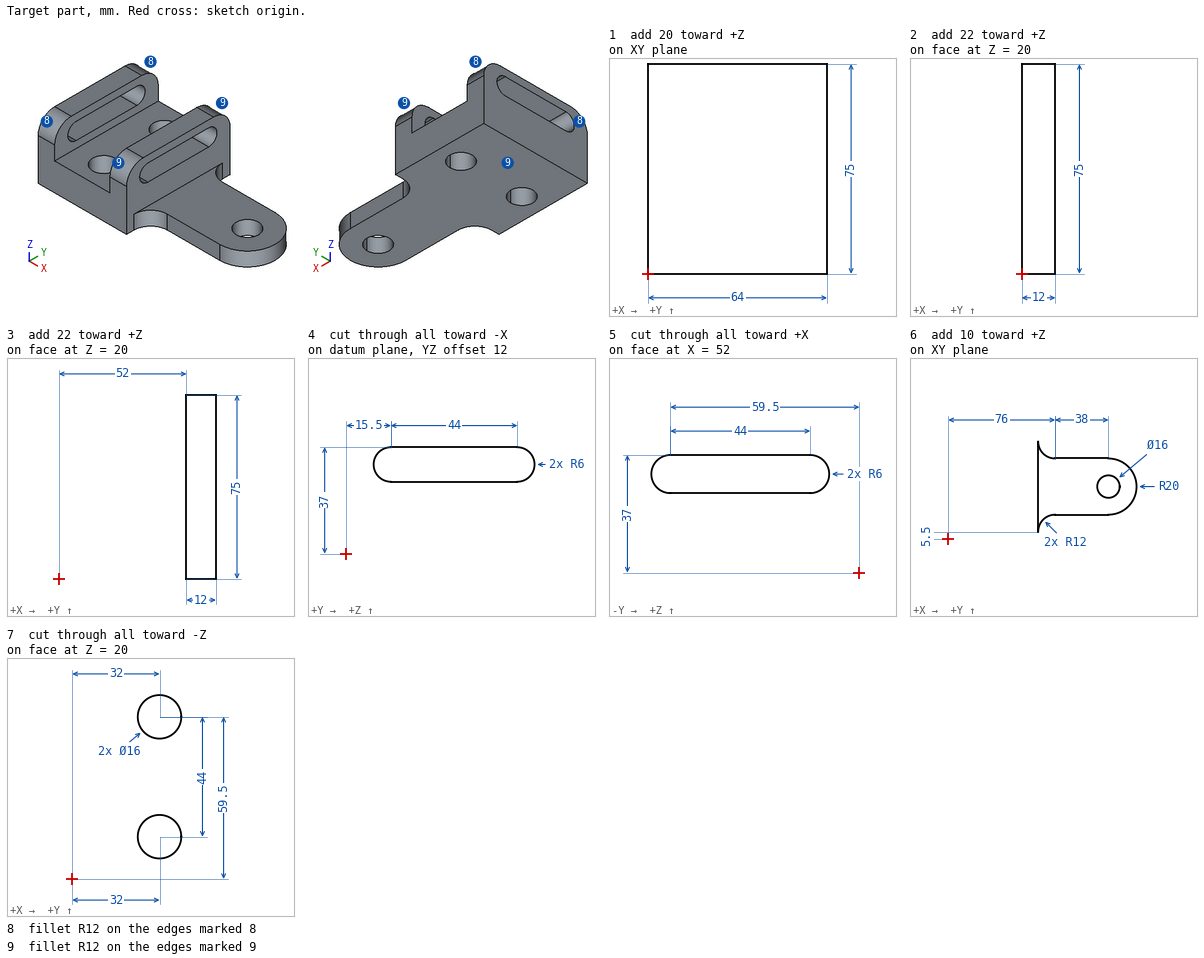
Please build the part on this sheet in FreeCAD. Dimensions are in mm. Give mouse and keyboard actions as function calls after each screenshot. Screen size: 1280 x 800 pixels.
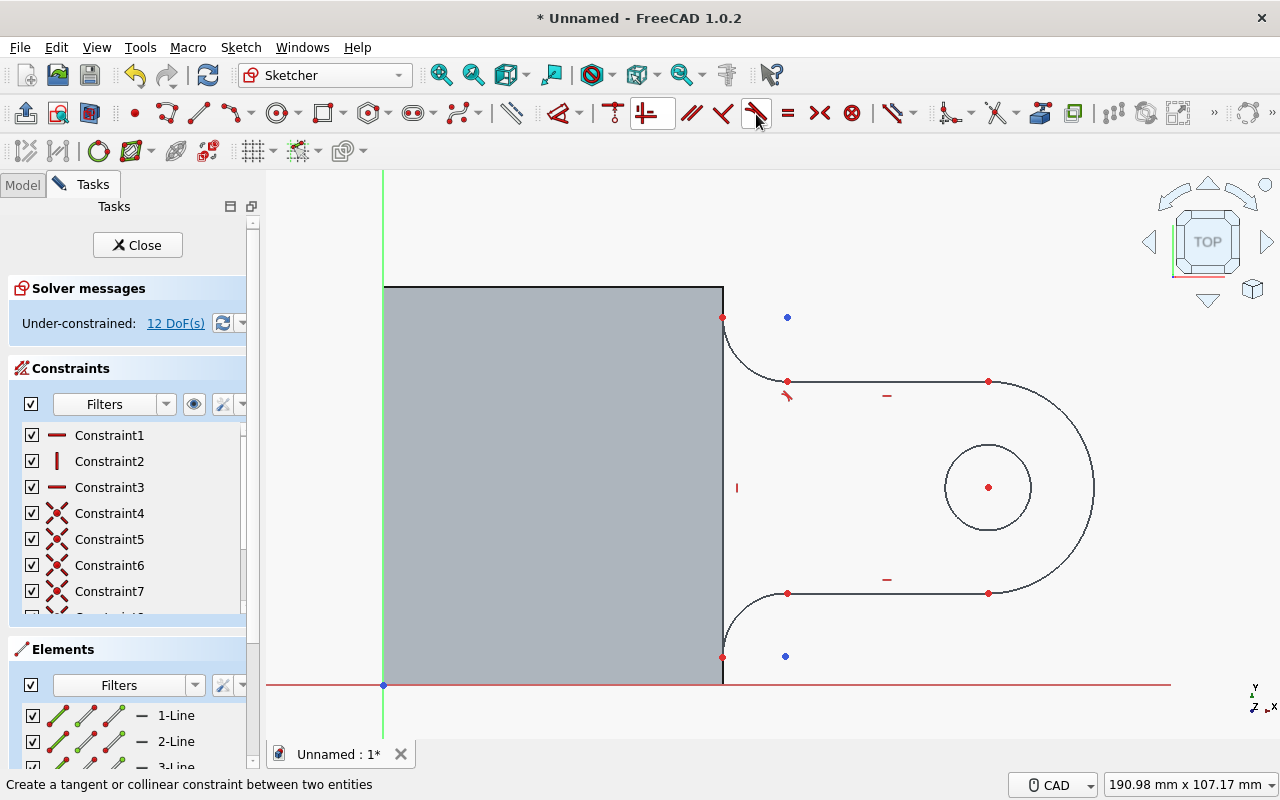
click(928, 382)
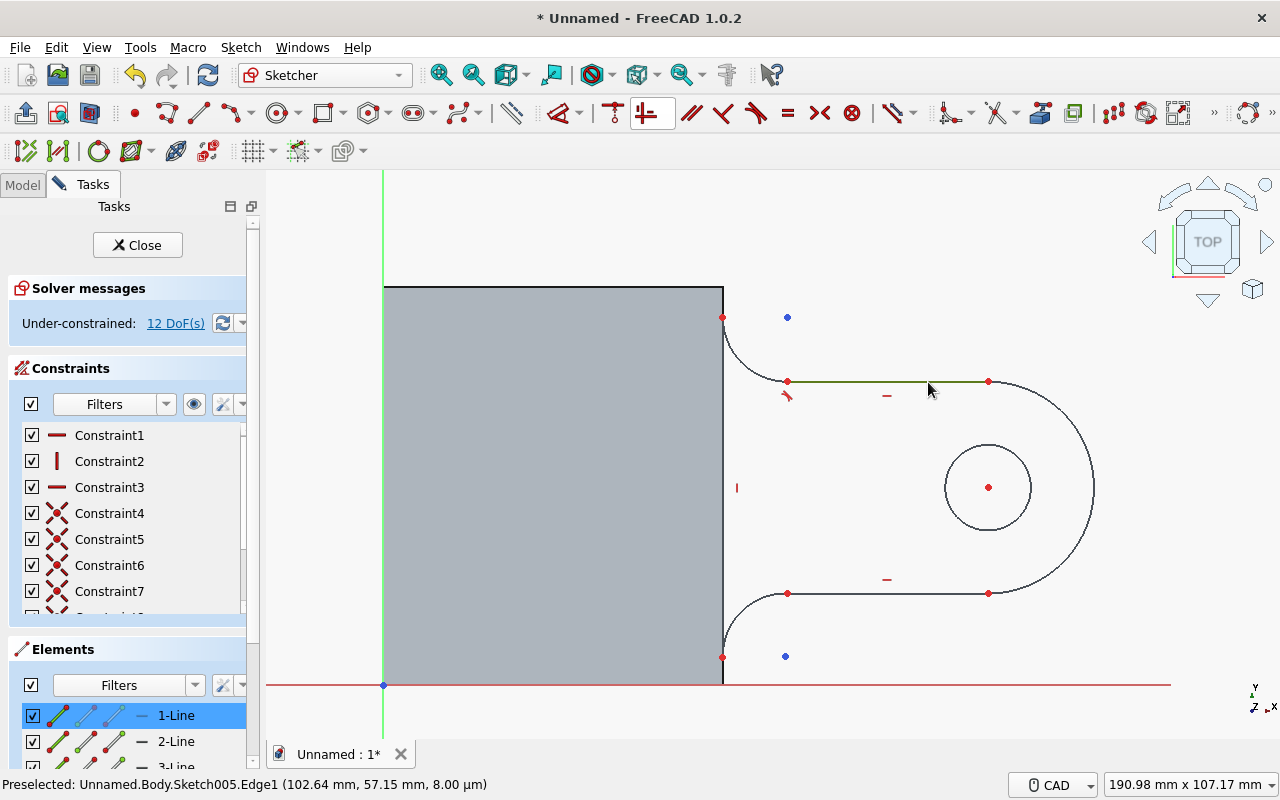
click(1074, 550)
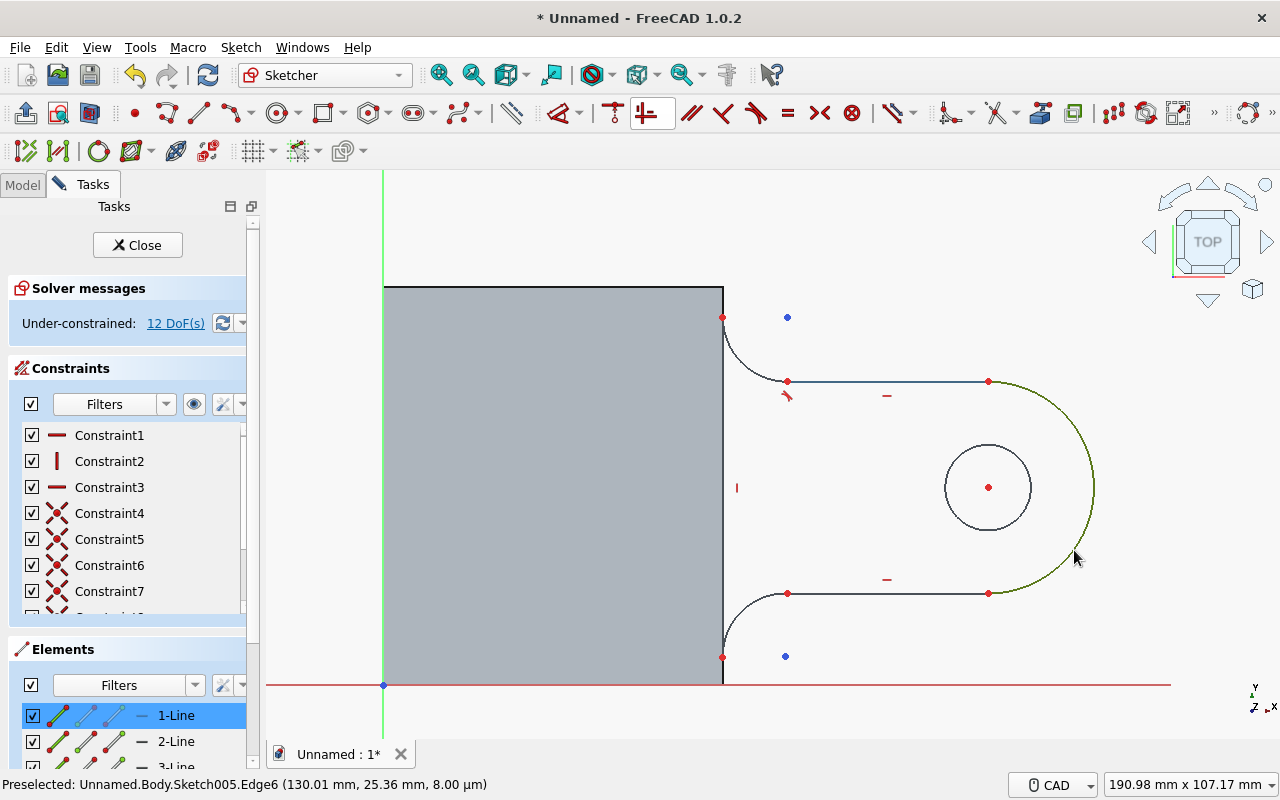
click(756, 114)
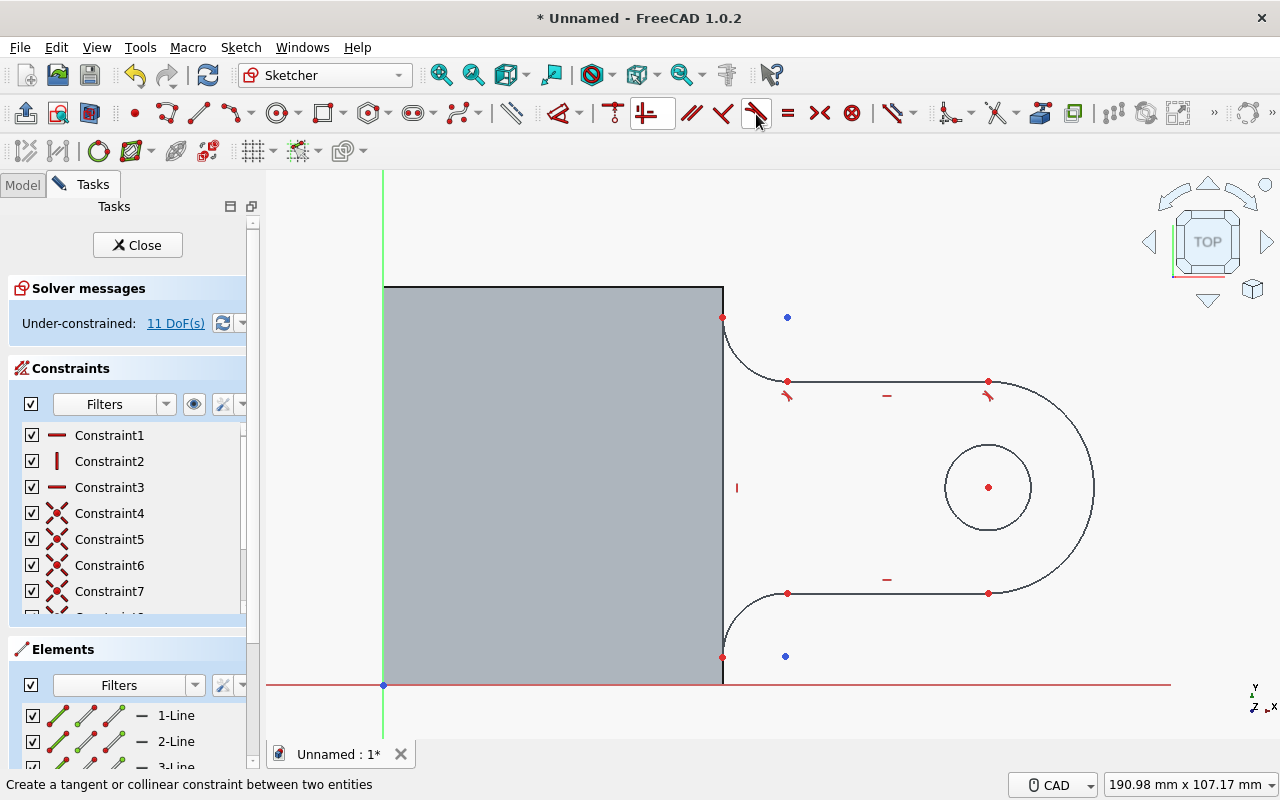
click(723, 420)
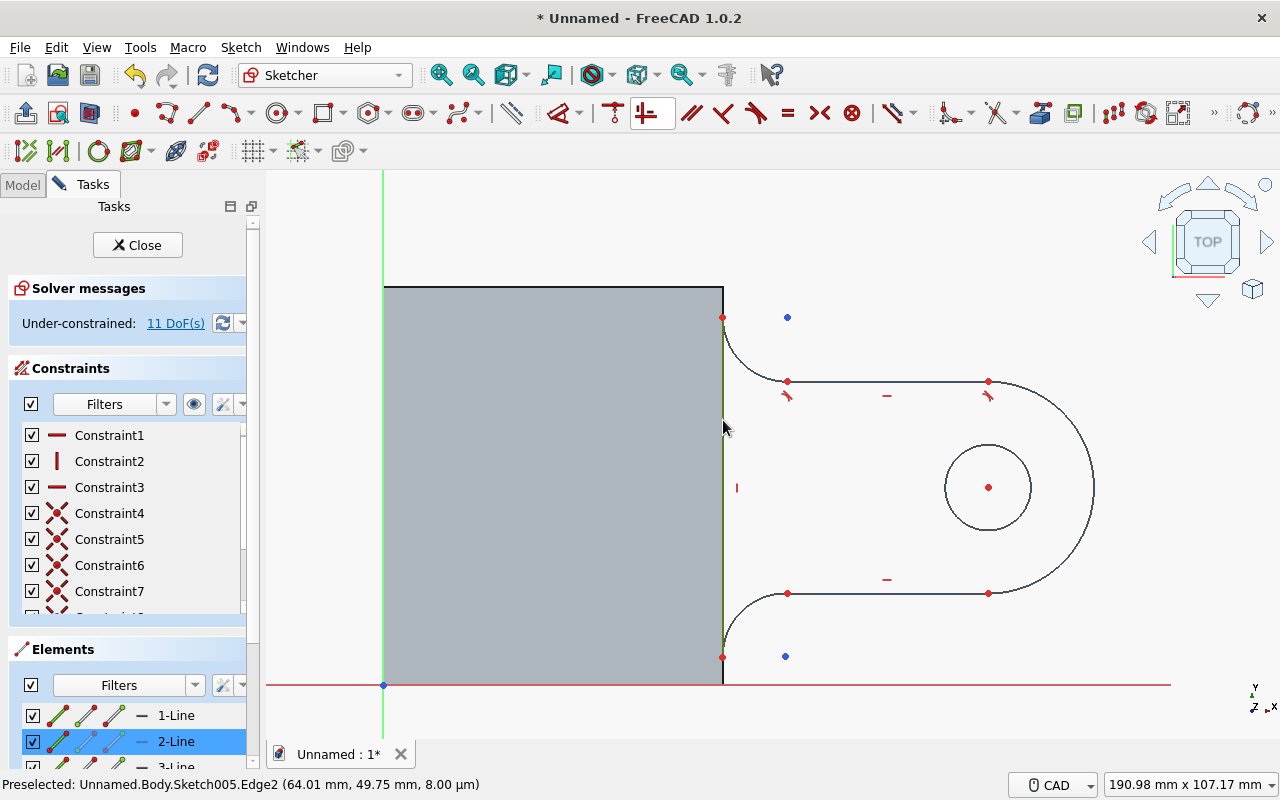
click(758, 375)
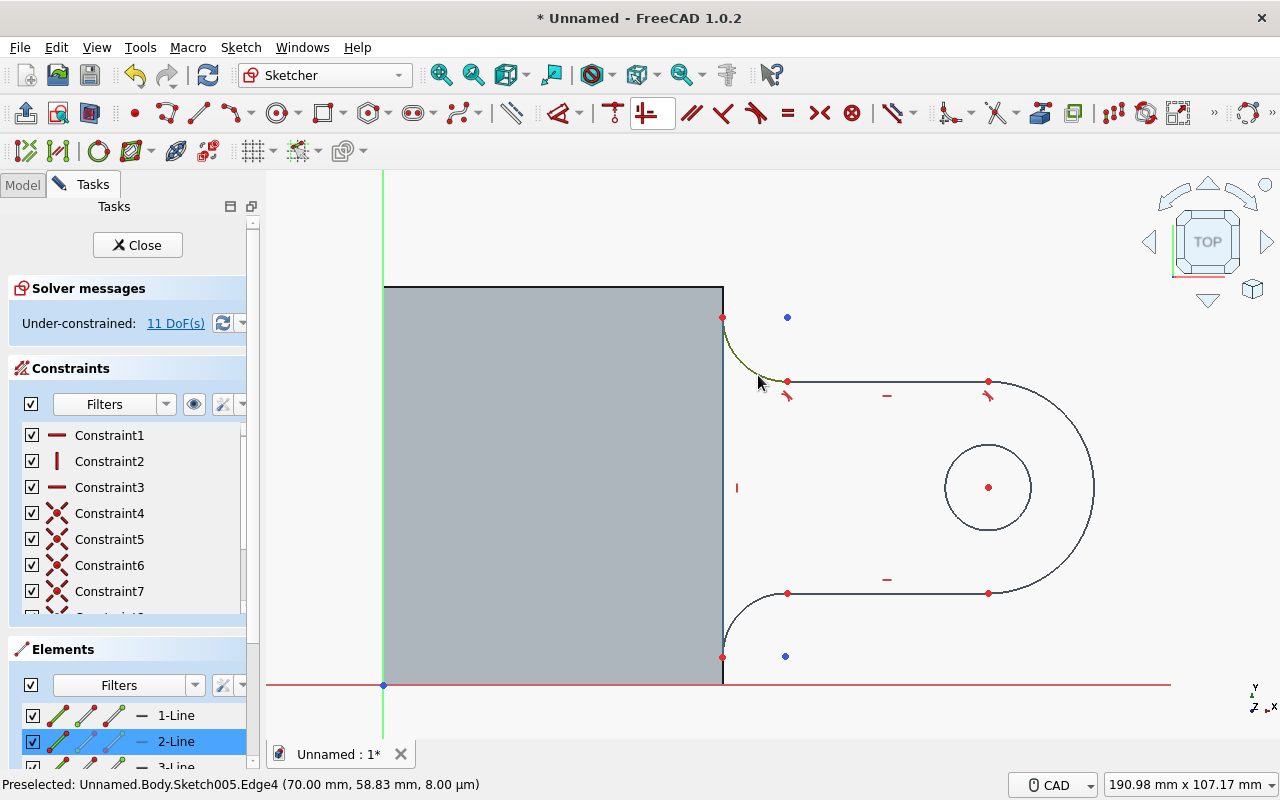
click(756, 114)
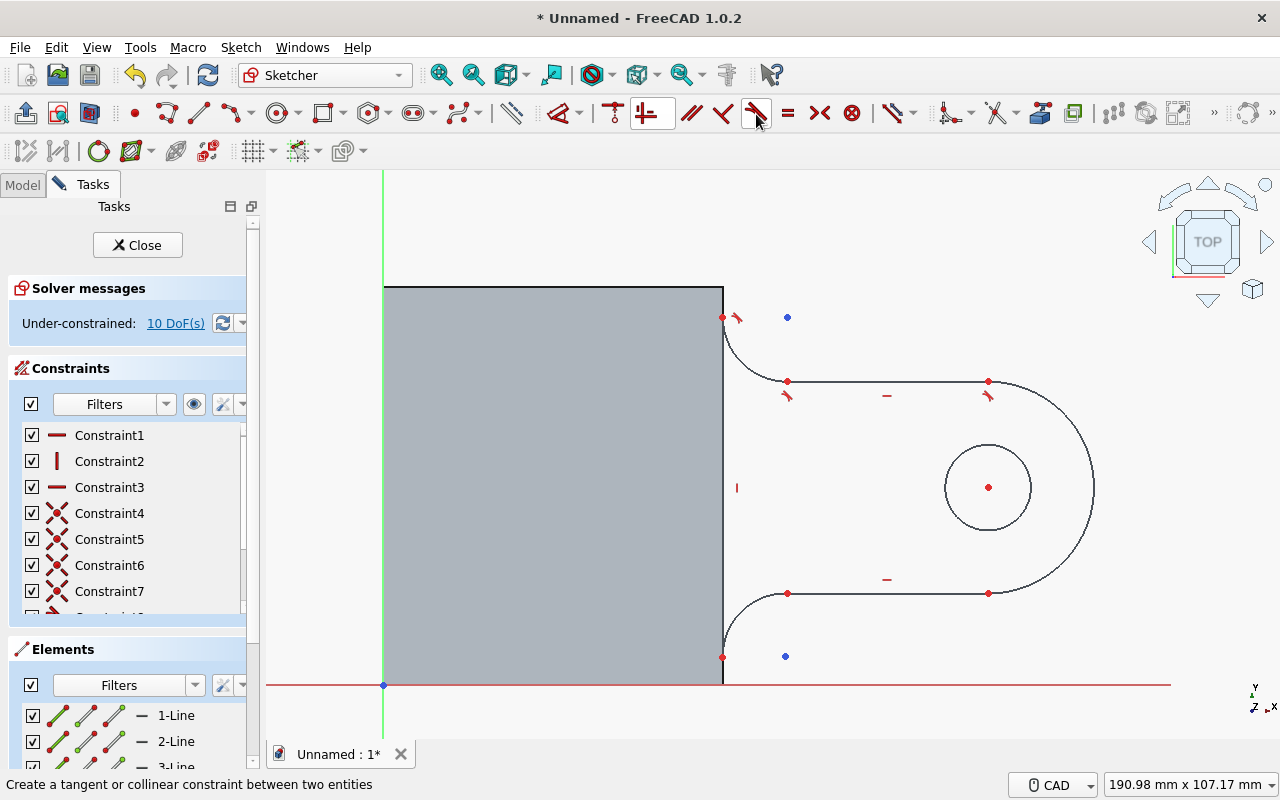
click(723, 419)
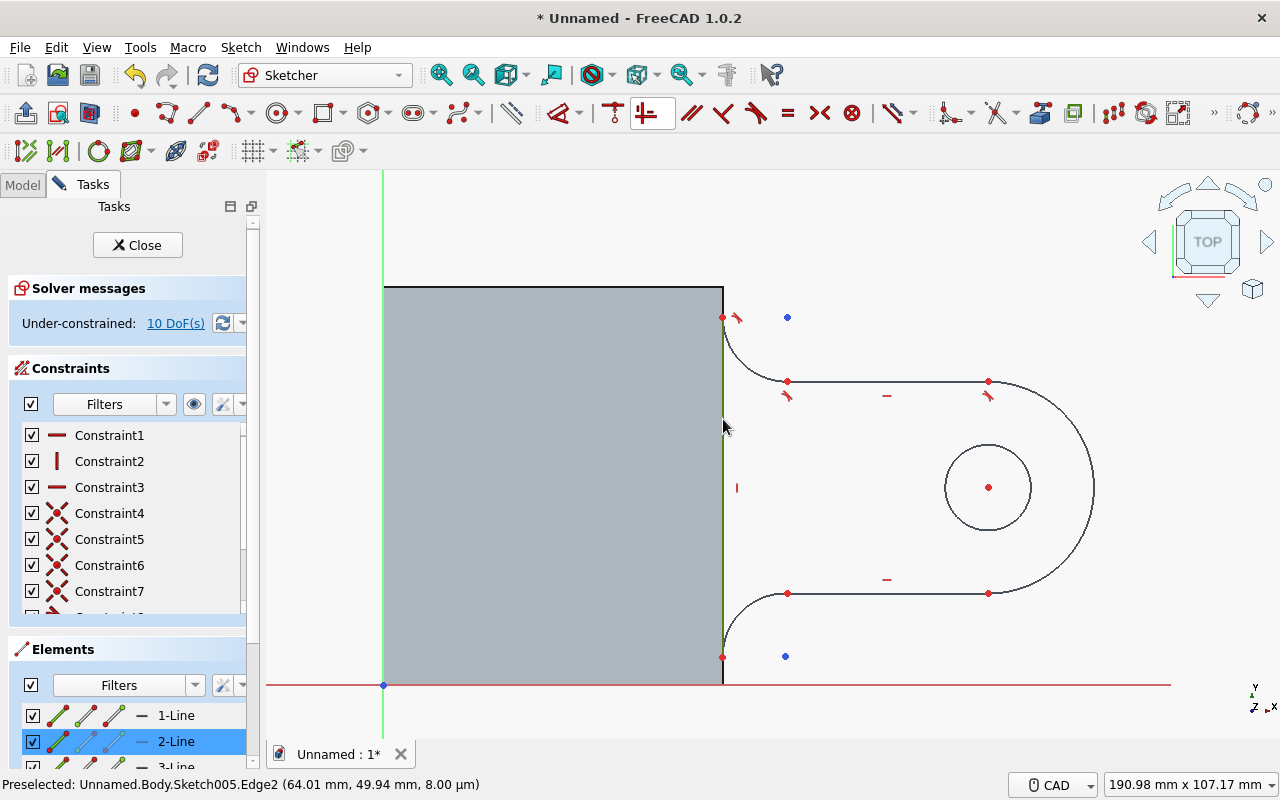
click(758, 600)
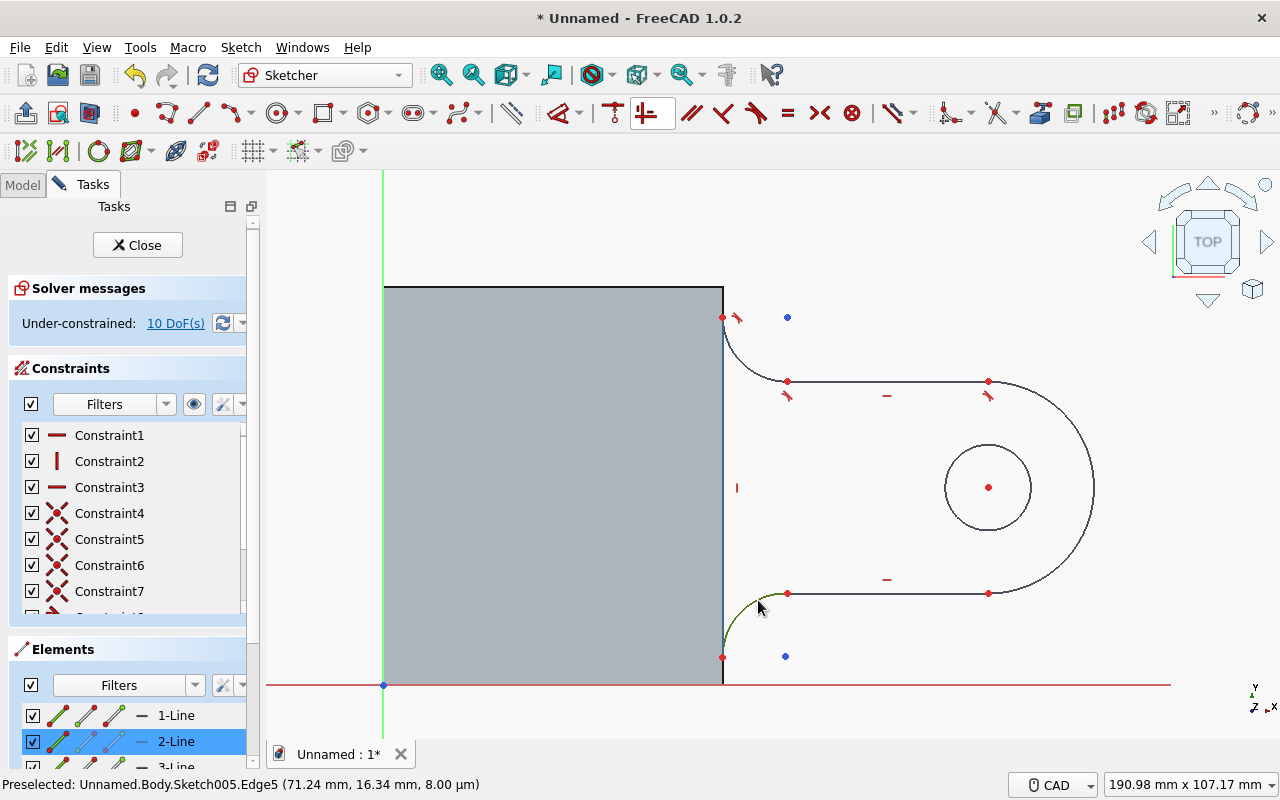
click(756, 114)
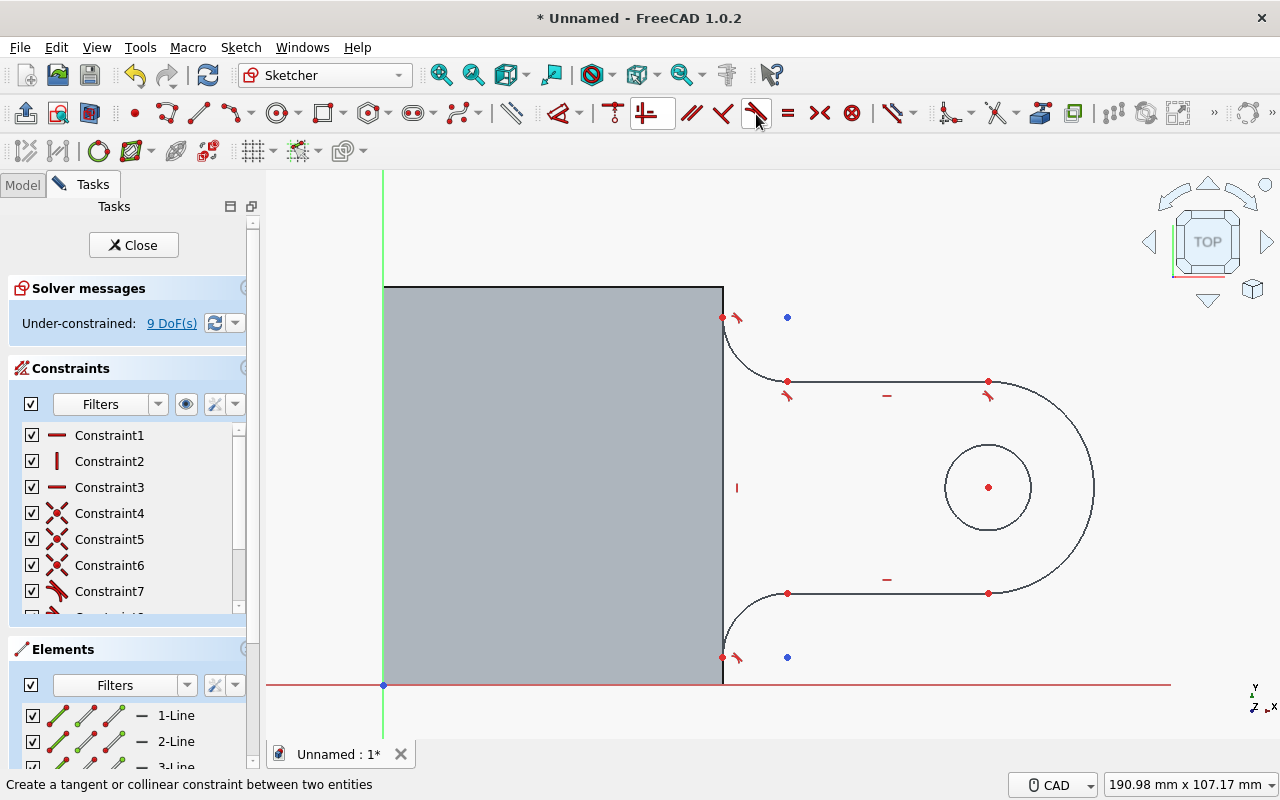
click(847, 594)